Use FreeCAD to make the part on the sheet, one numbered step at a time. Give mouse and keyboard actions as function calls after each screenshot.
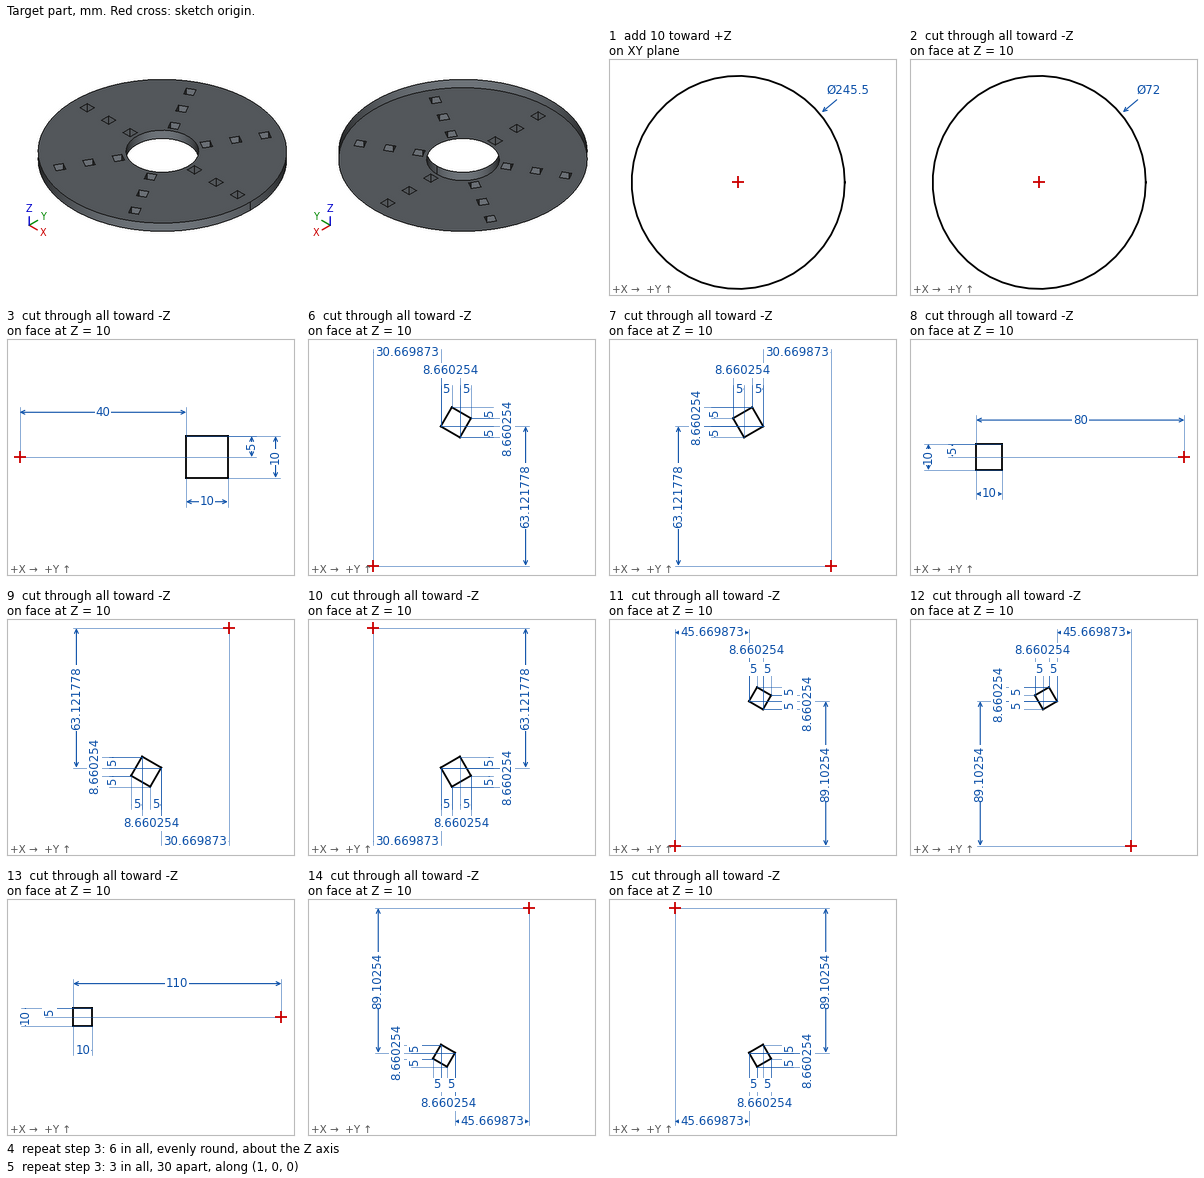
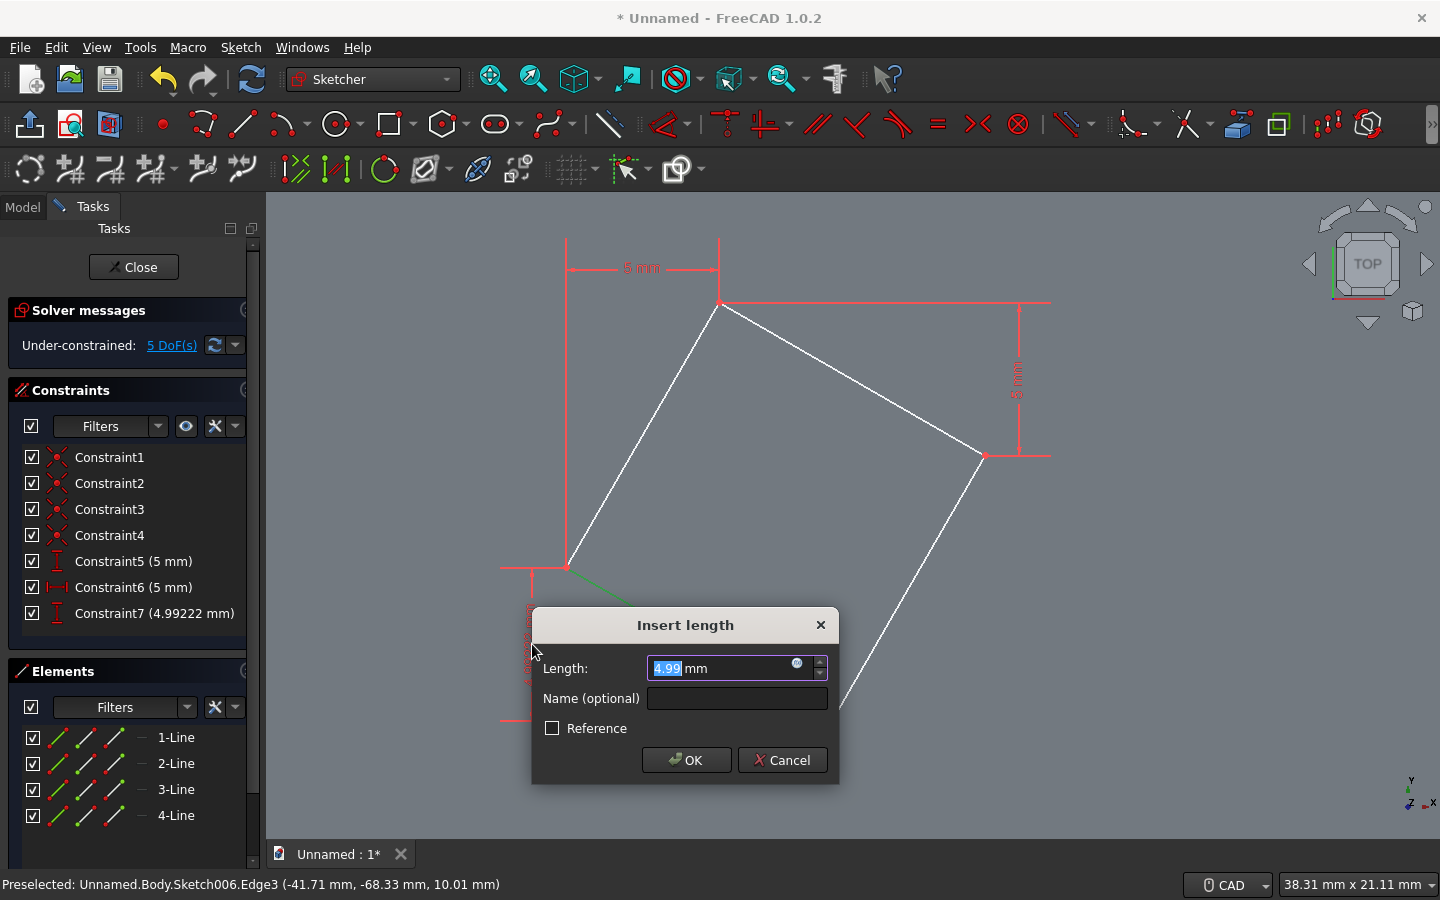
text(5)
key(Return)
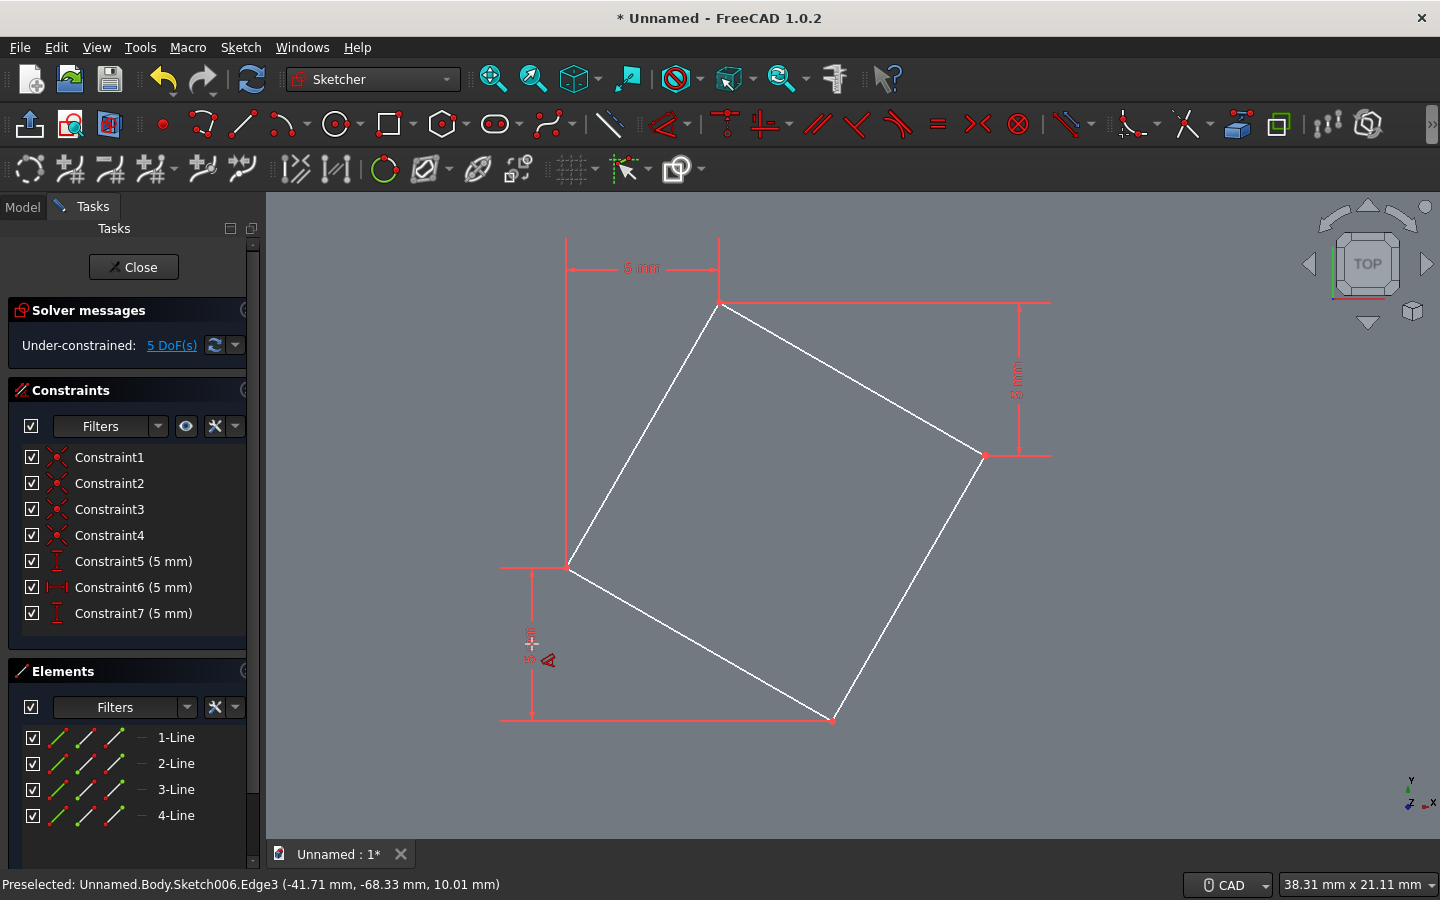
click(878, 642)
click(908, 755)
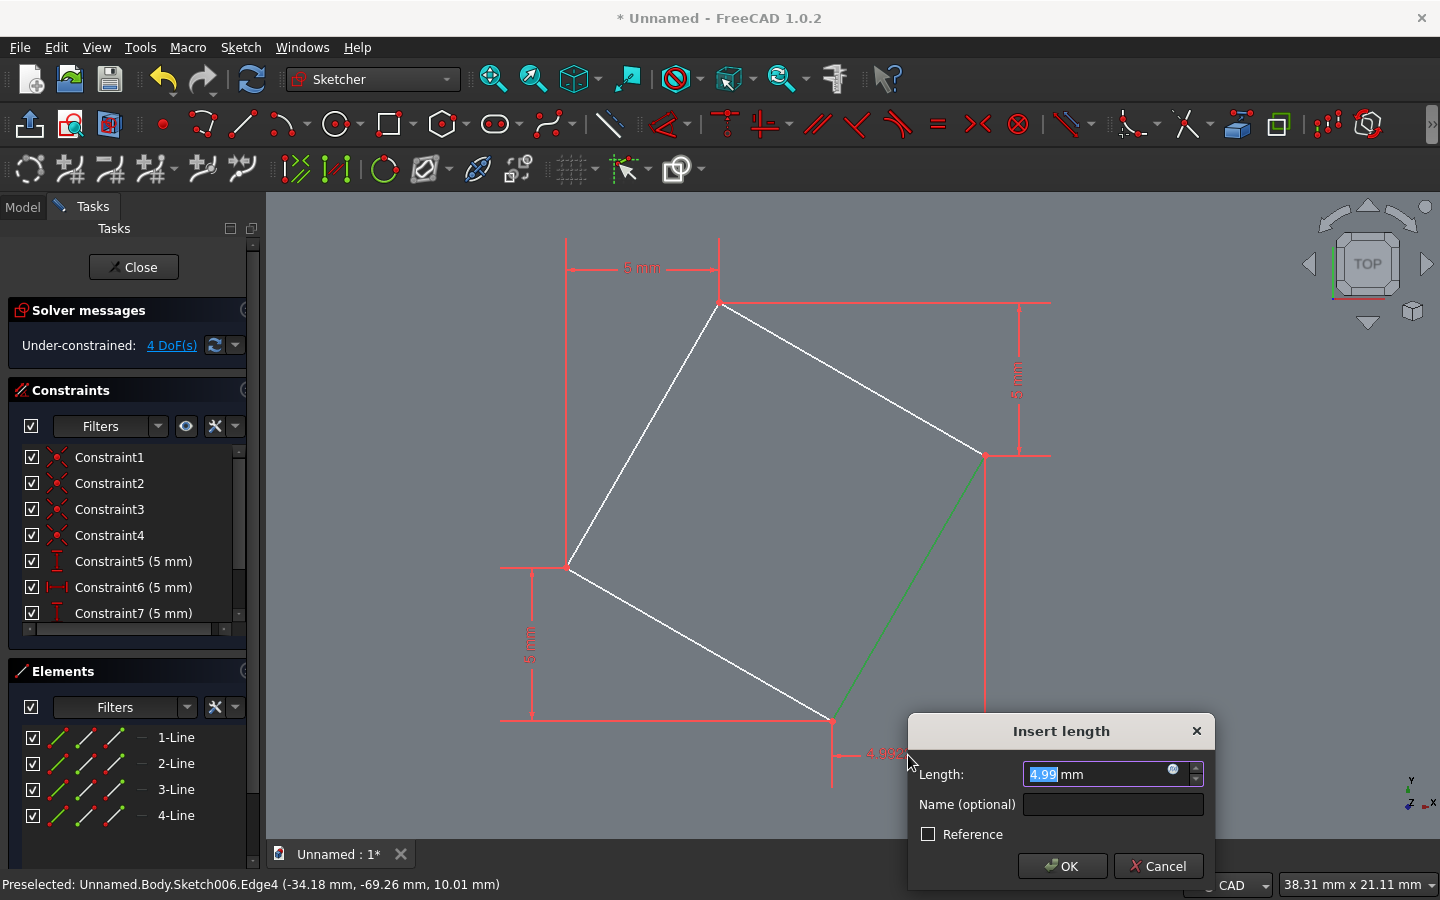
text(5)
key(Return)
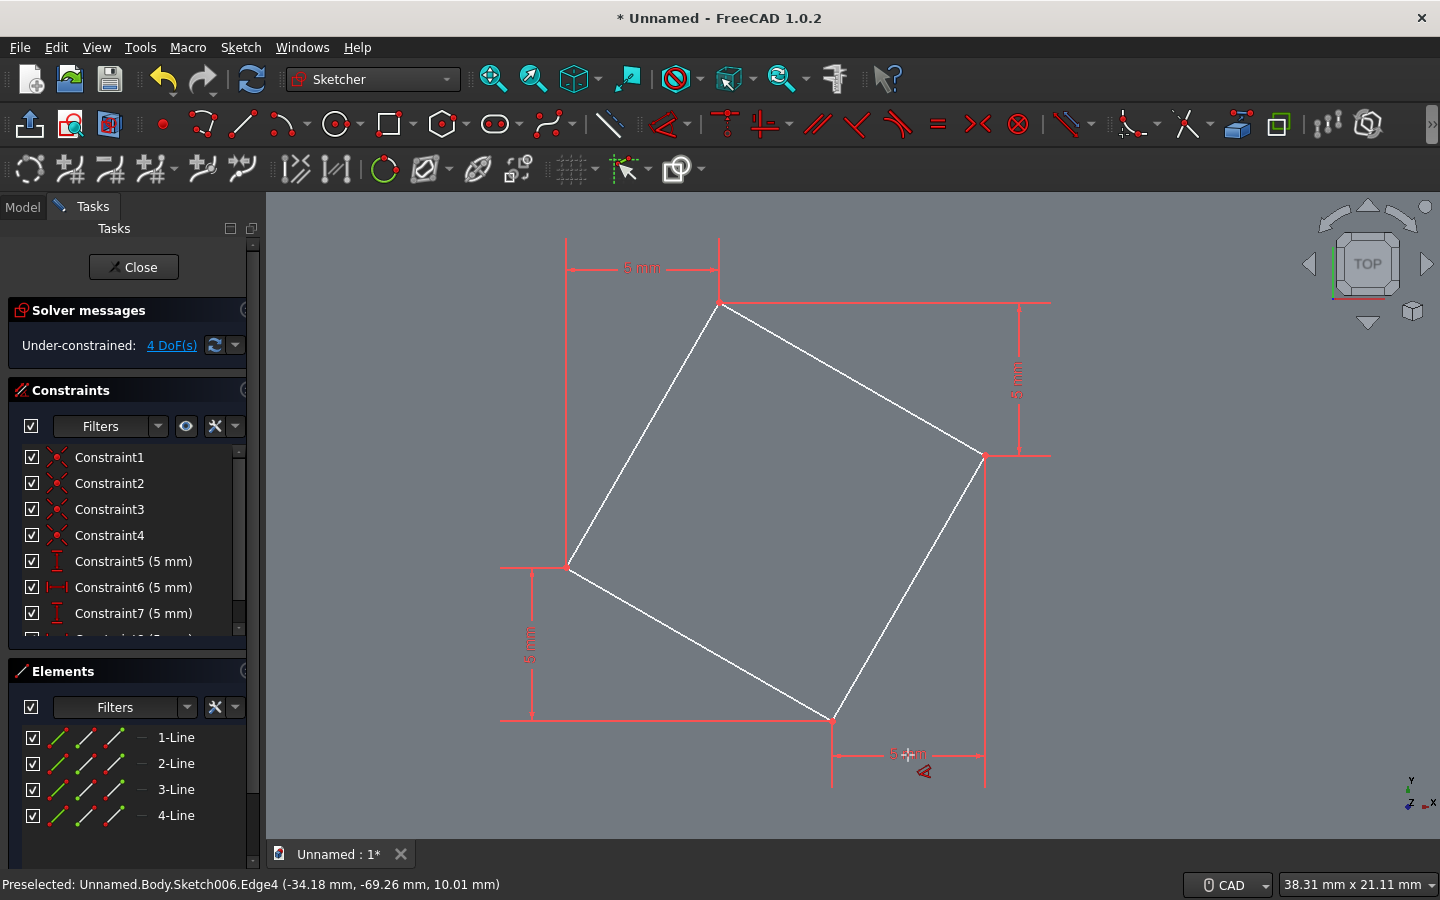
click(905, 410)
click(852, 269)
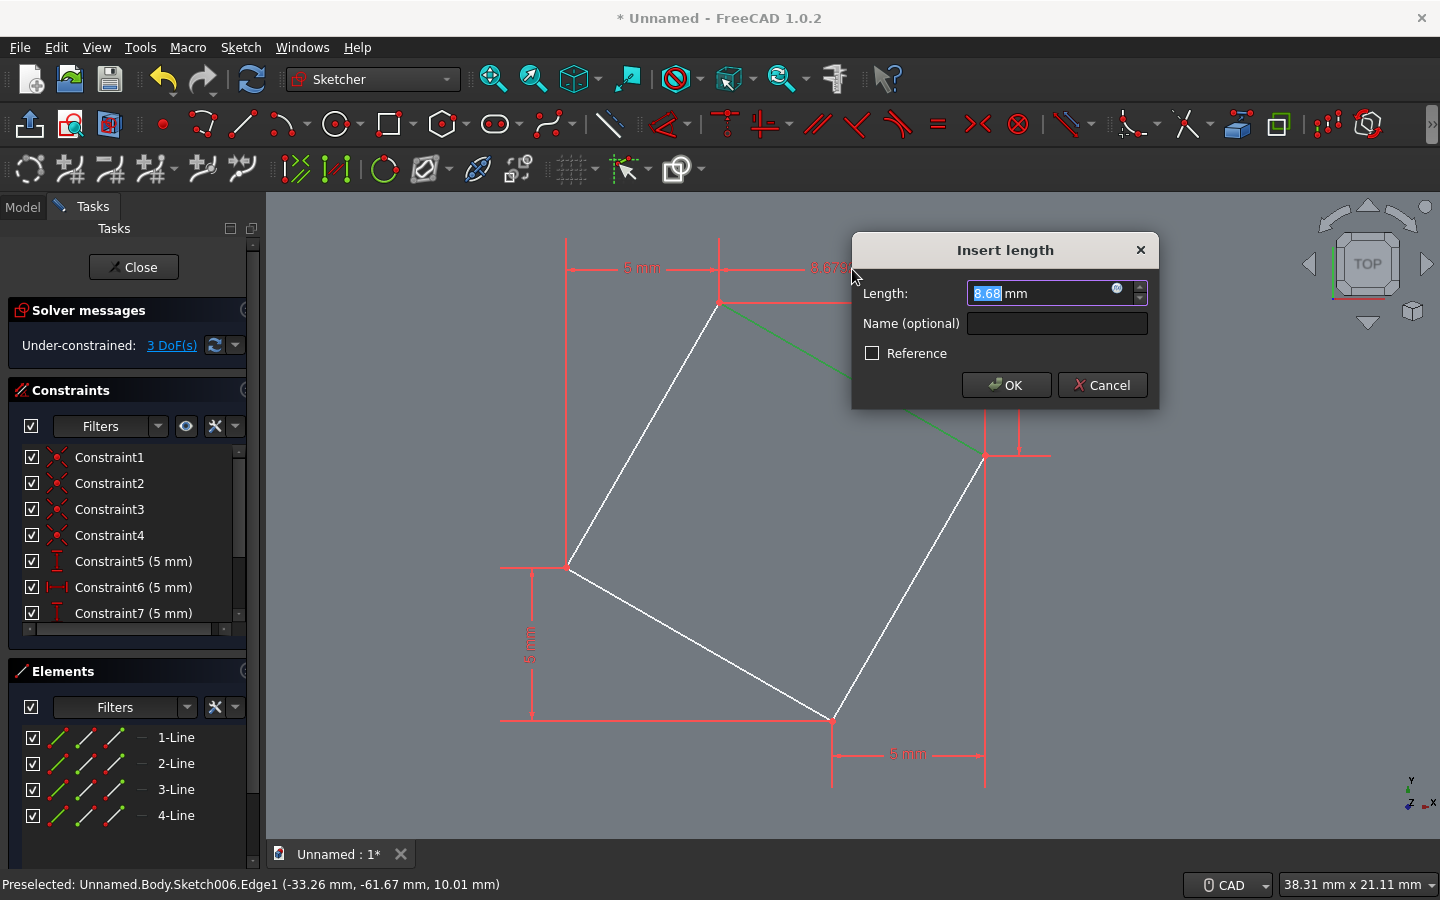
text(8.660254)
key(Return)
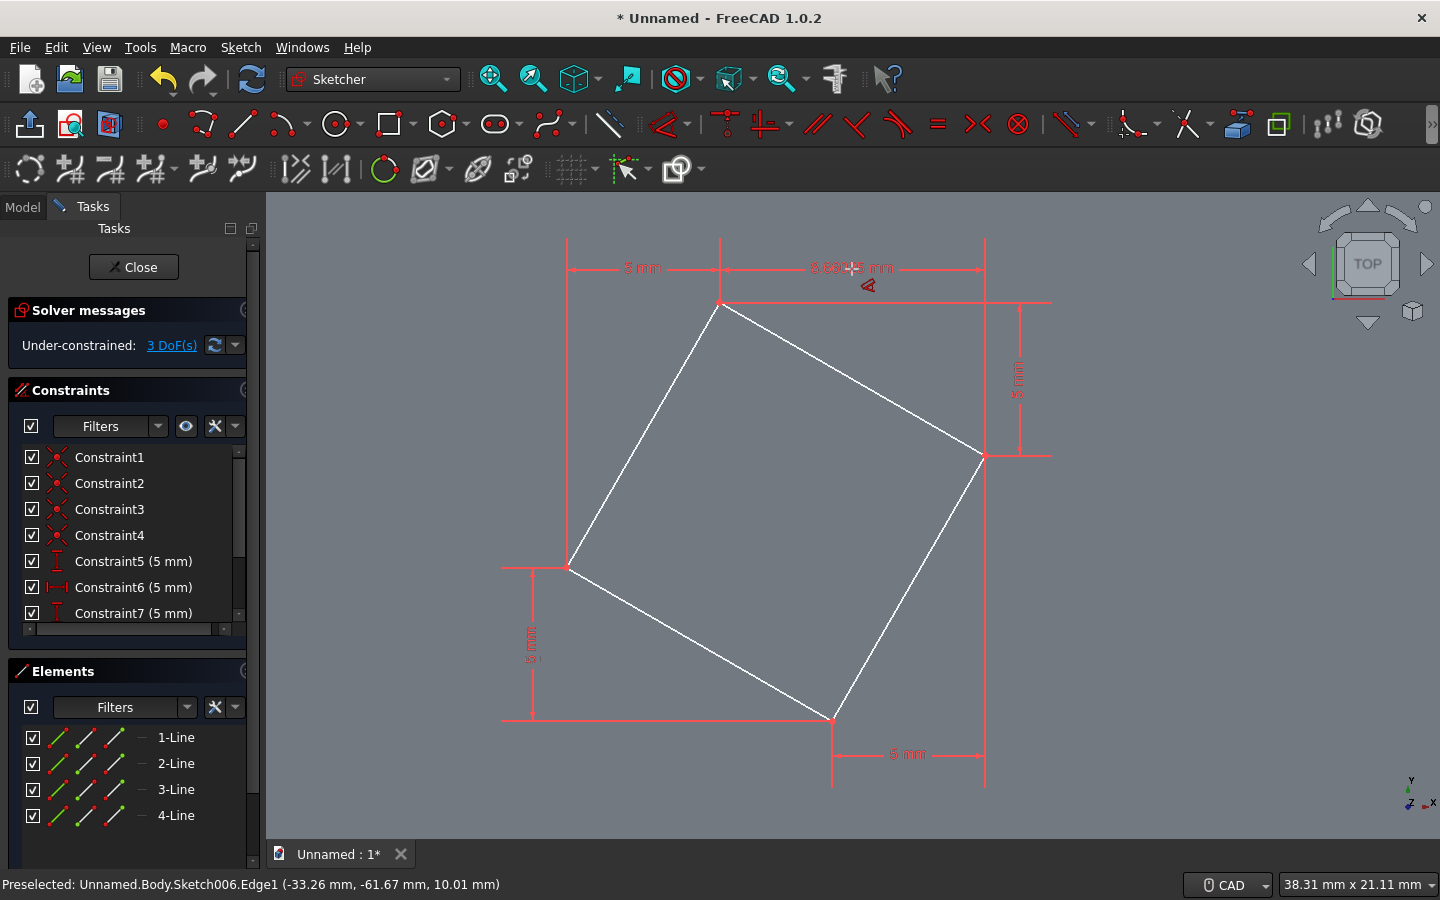
click(674, 382)
click(533, 435)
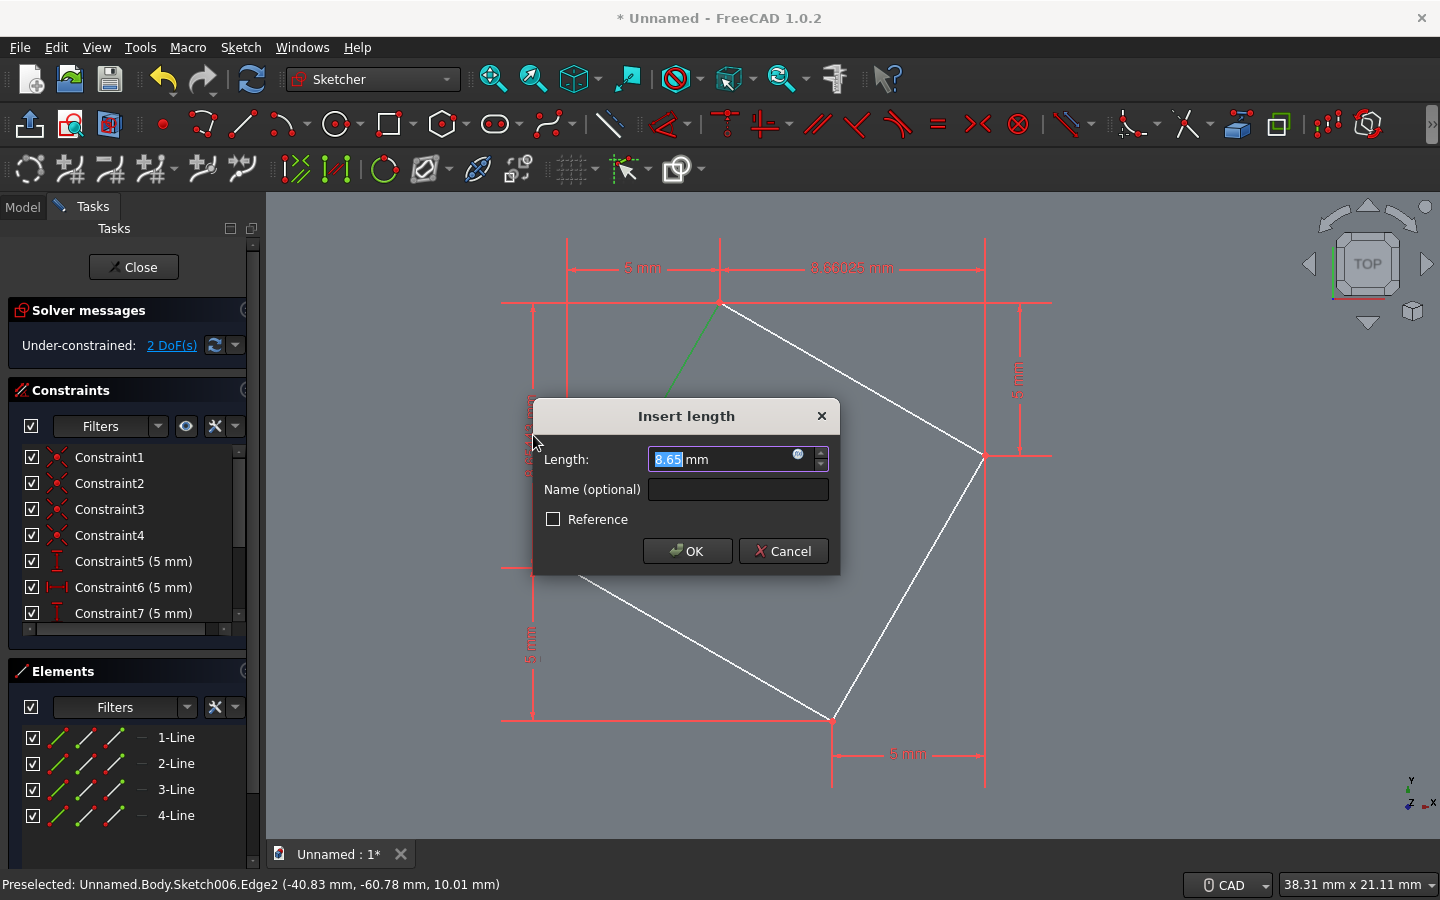
text(8.660254)
key(Return)